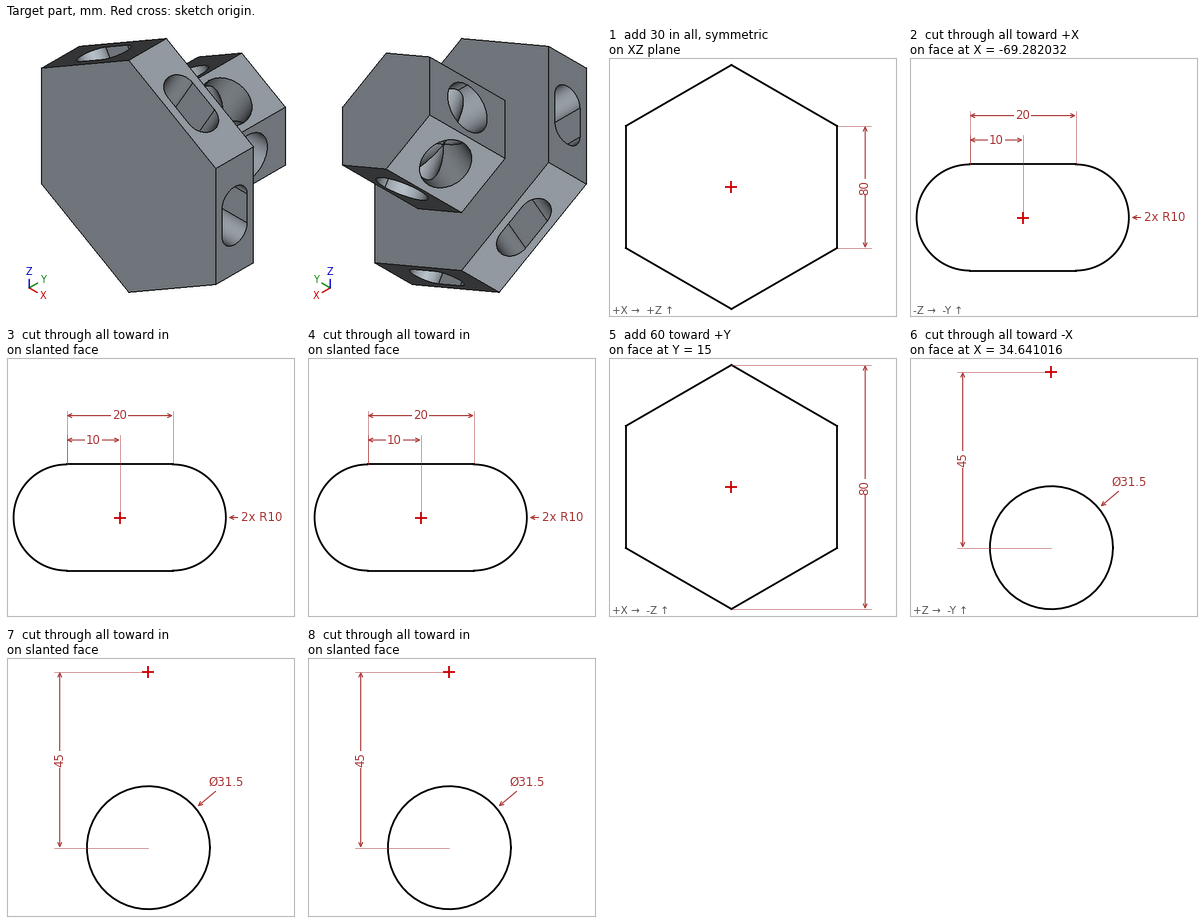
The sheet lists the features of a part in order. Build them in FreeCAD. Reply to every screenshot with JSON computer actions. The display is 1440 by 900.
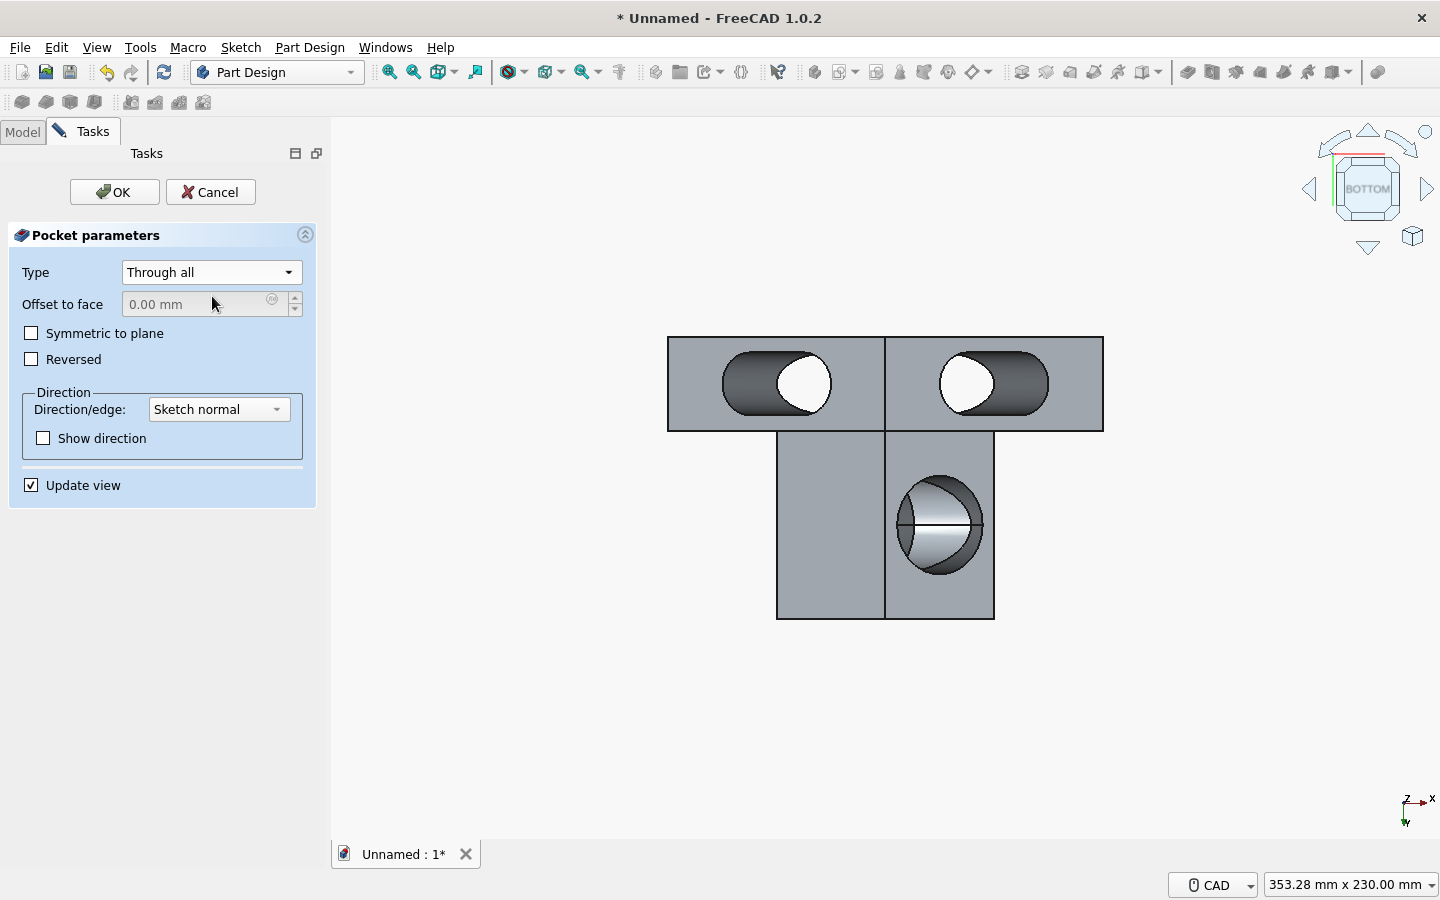
{"action": "left_click", "coordinate": [115, 192]}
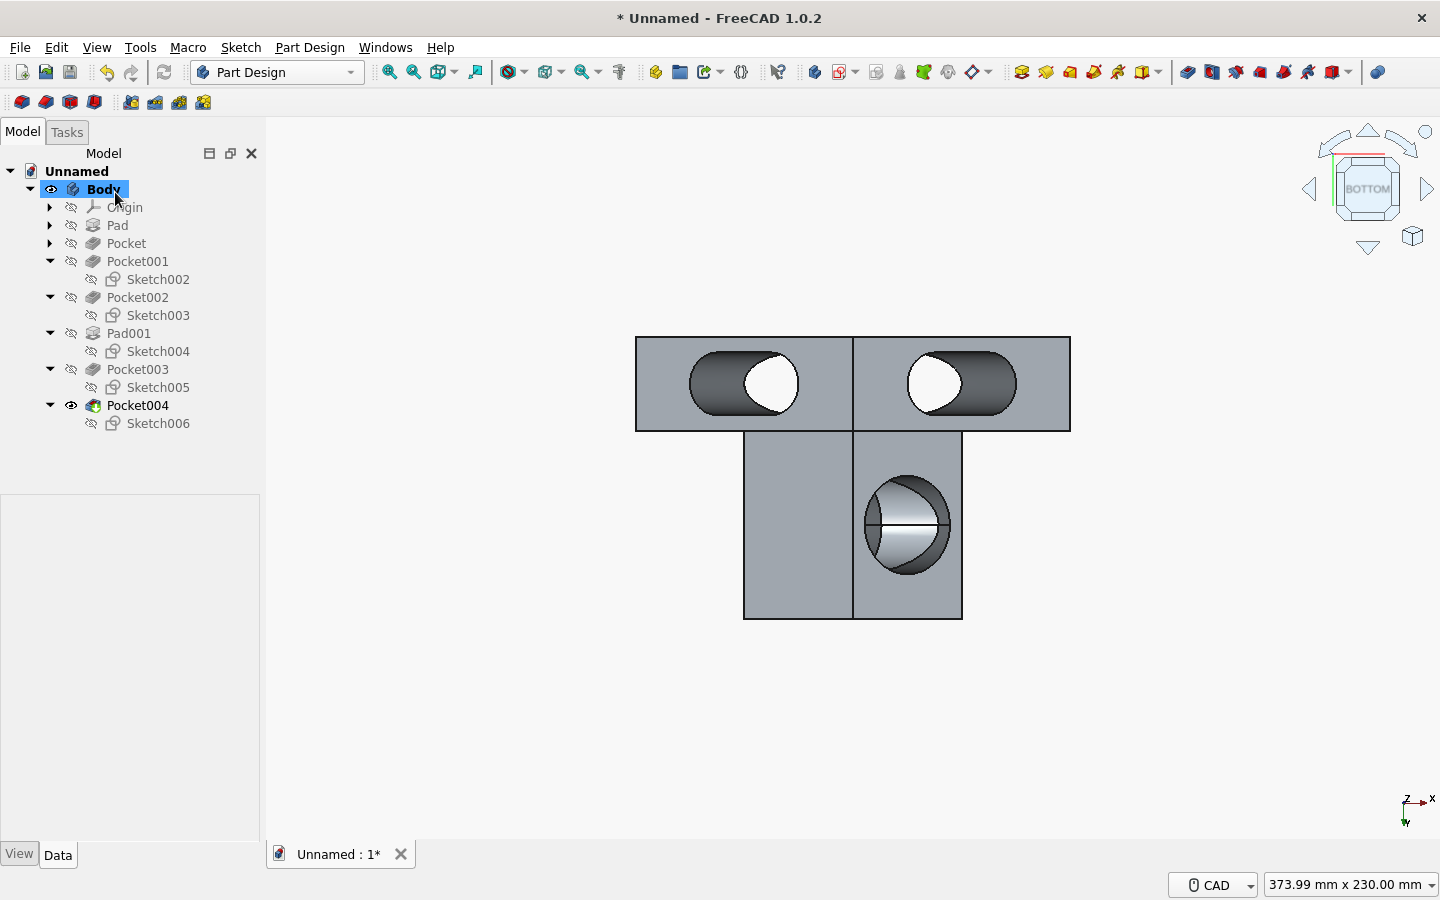
{"action": "left_click", "coordinate": [390, 72]}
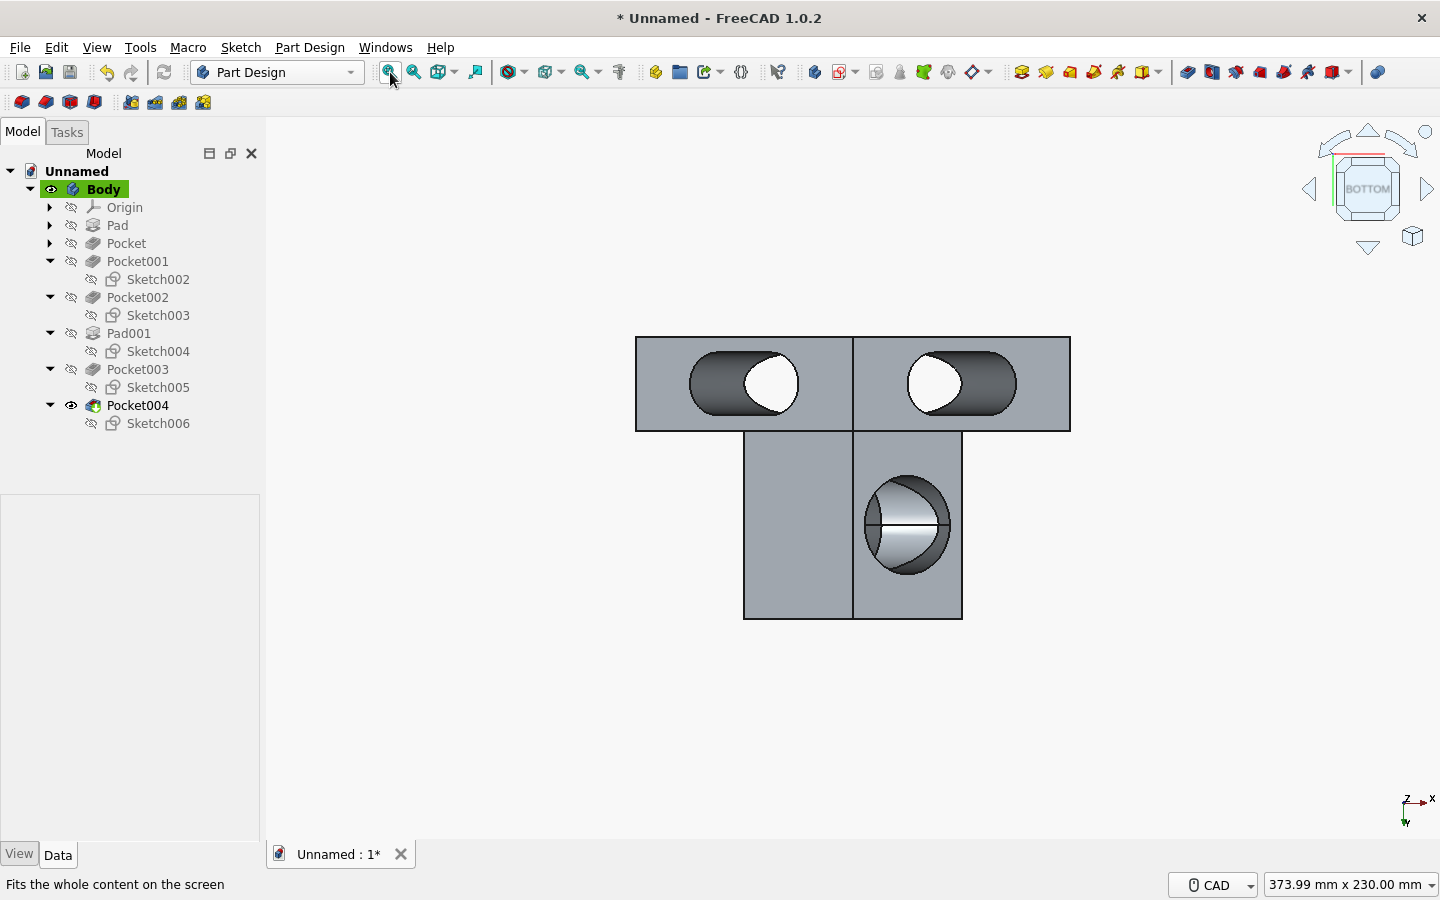
{"action": "key", "text": "0"}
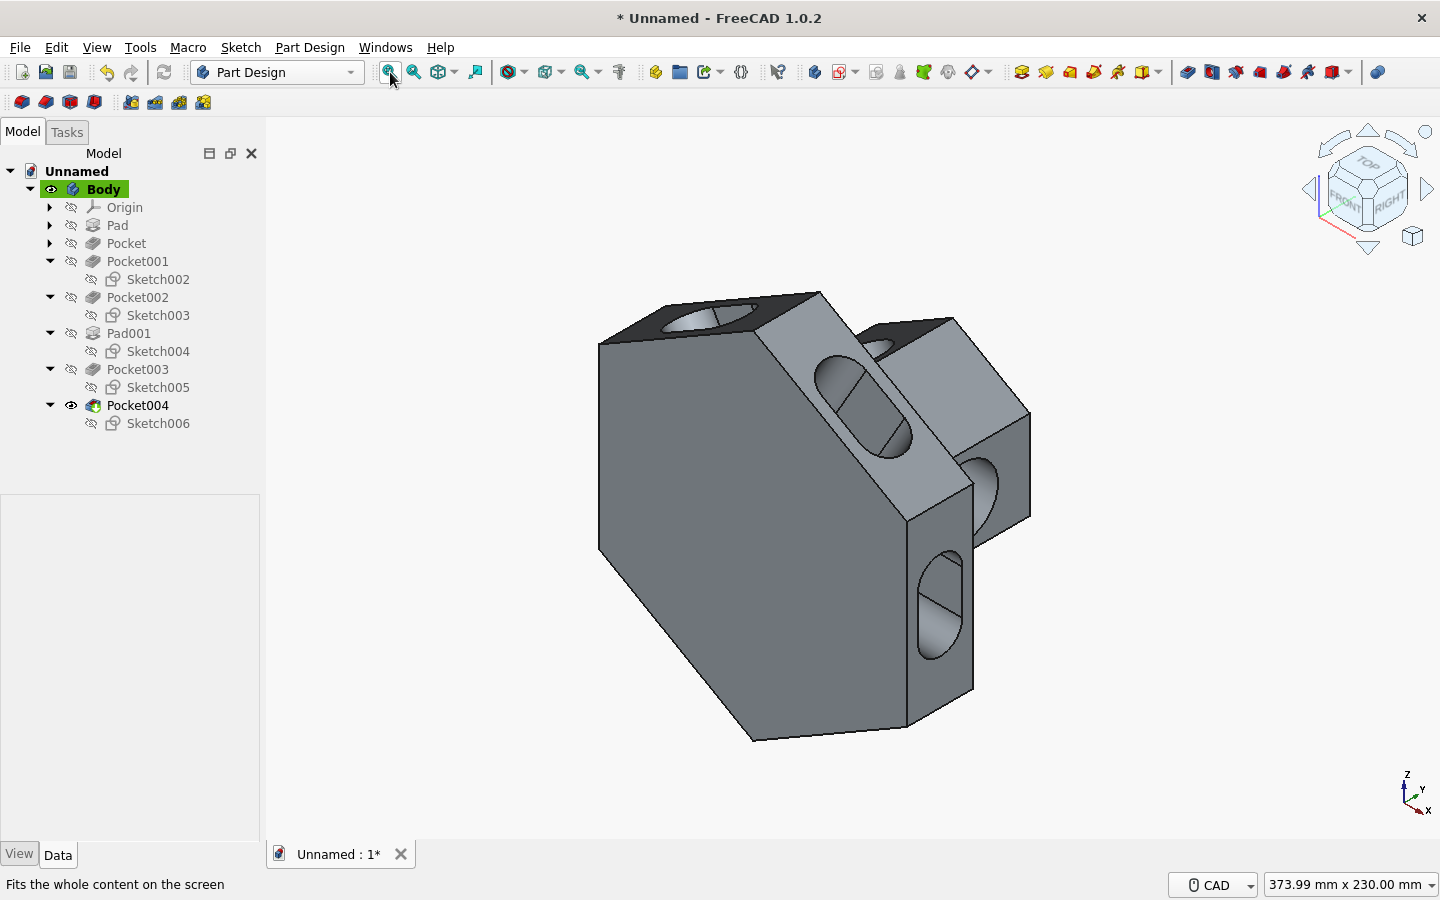
{"action": "left_click", "coordinate": [944, 392]}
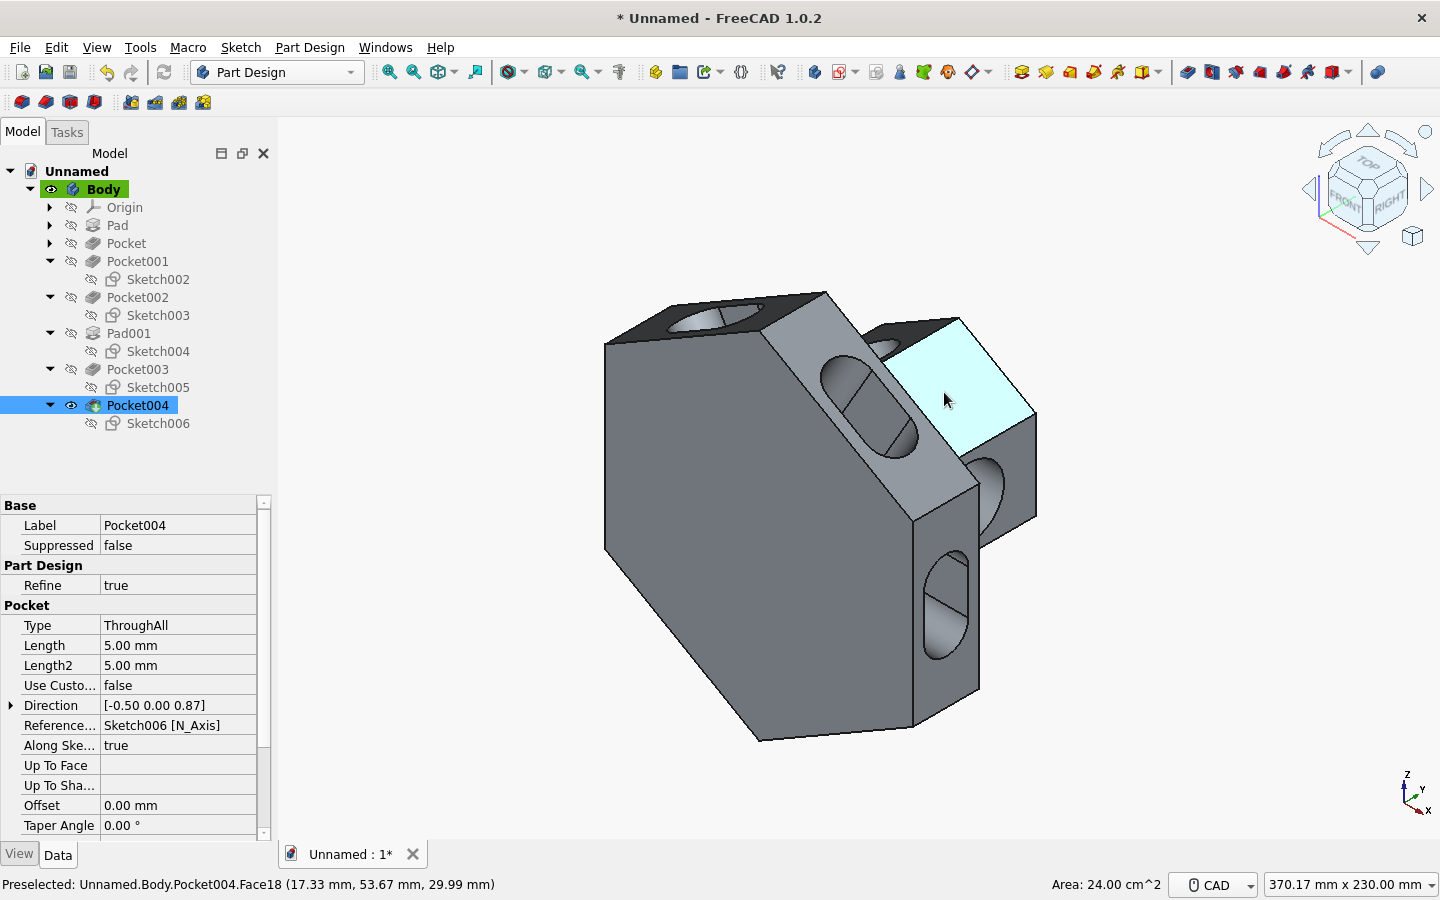
{"action": "left_click", "coordinate": [840, 72]}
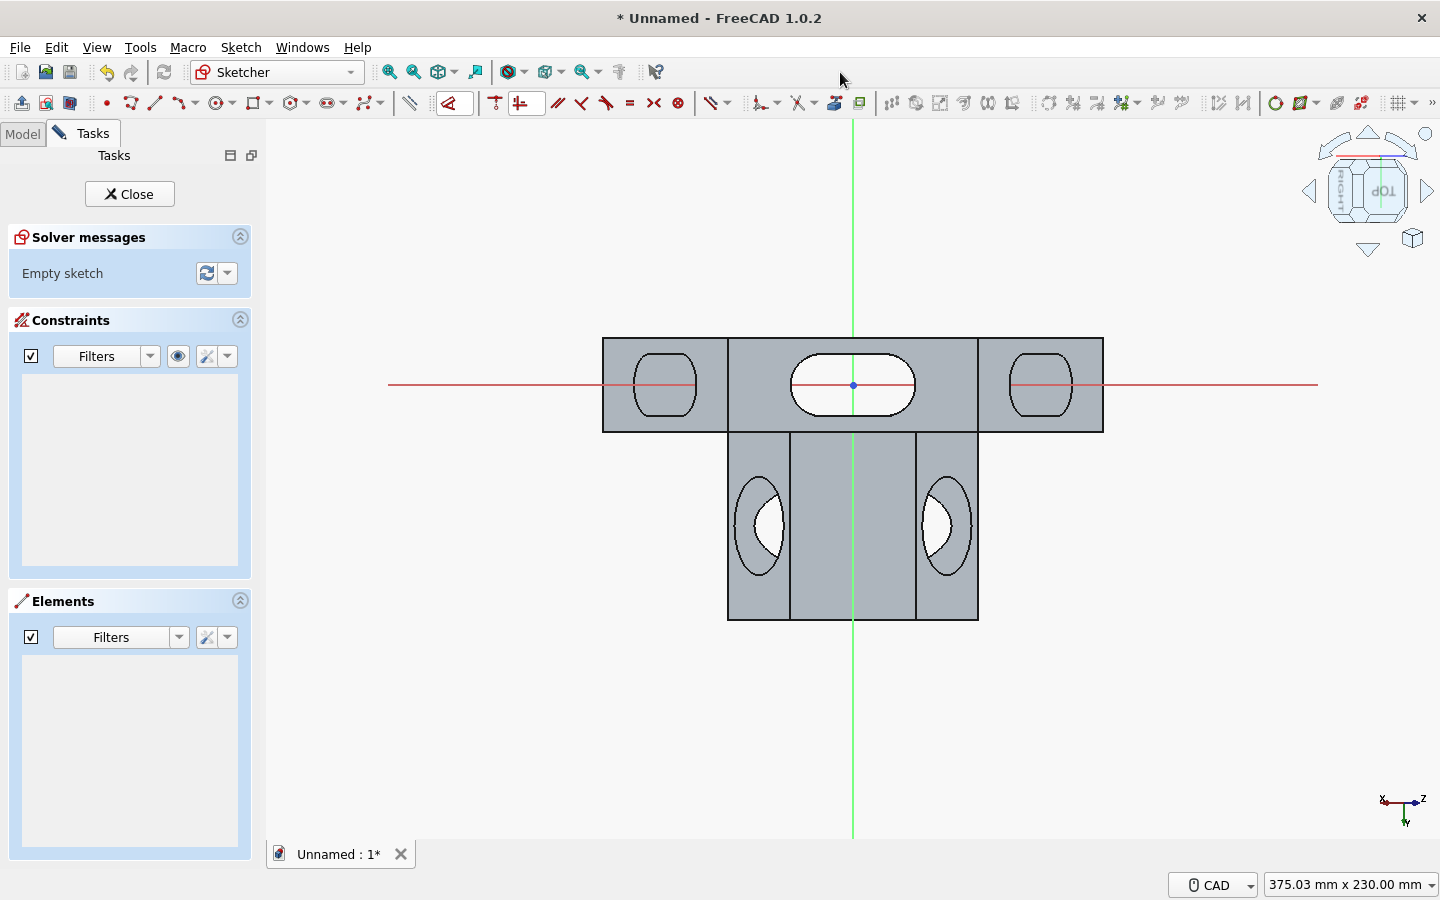
{"action": "scroll", "coordinate": [893, 481], "scroll_direction": "up", "scroll_amount": 5}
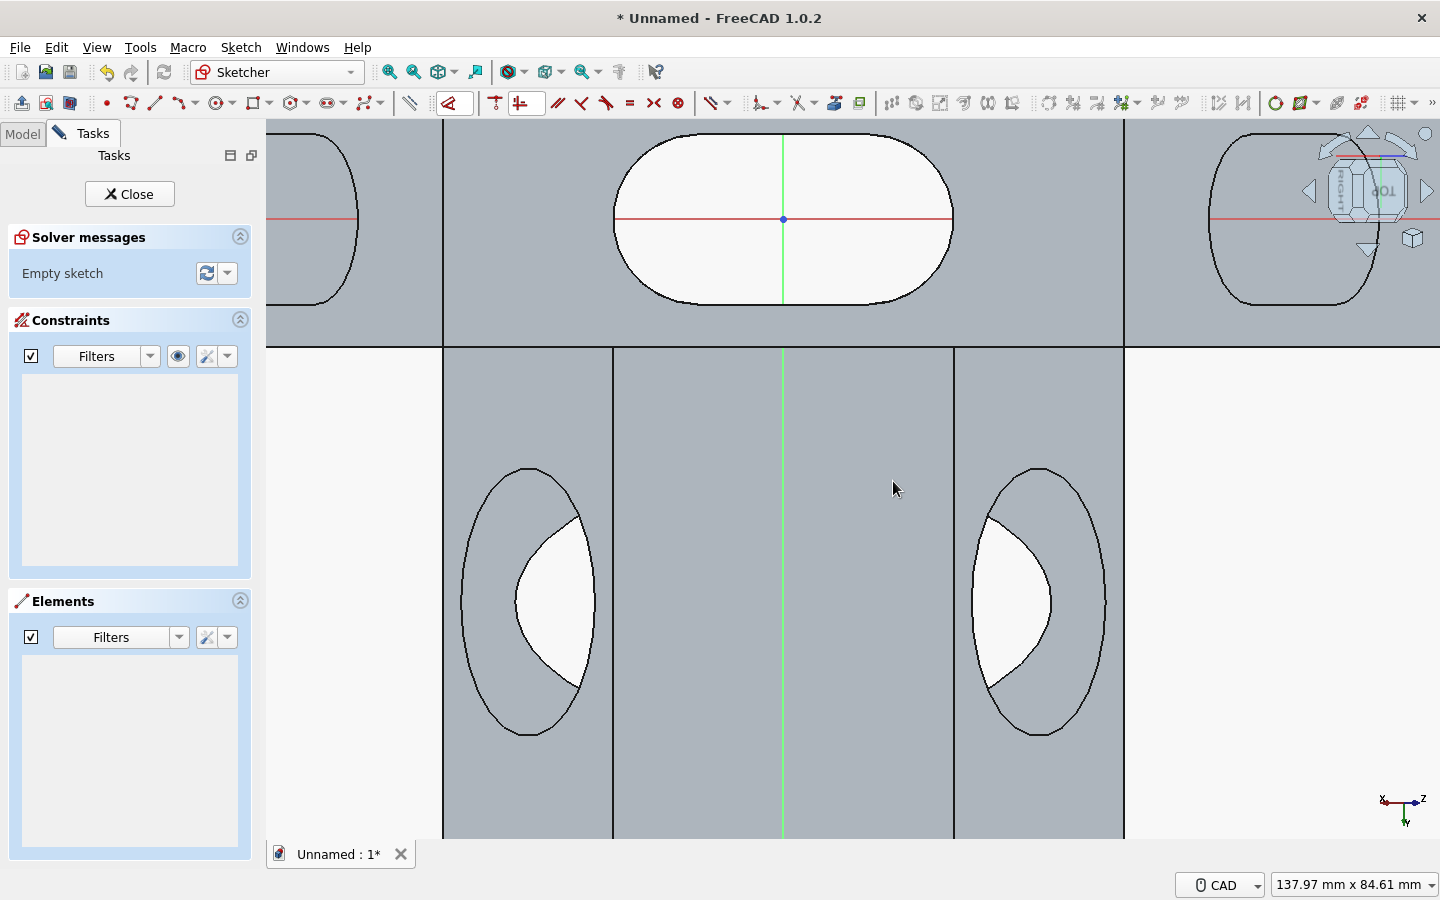
{"action": "left_click", "coordinate": [216, 104]}